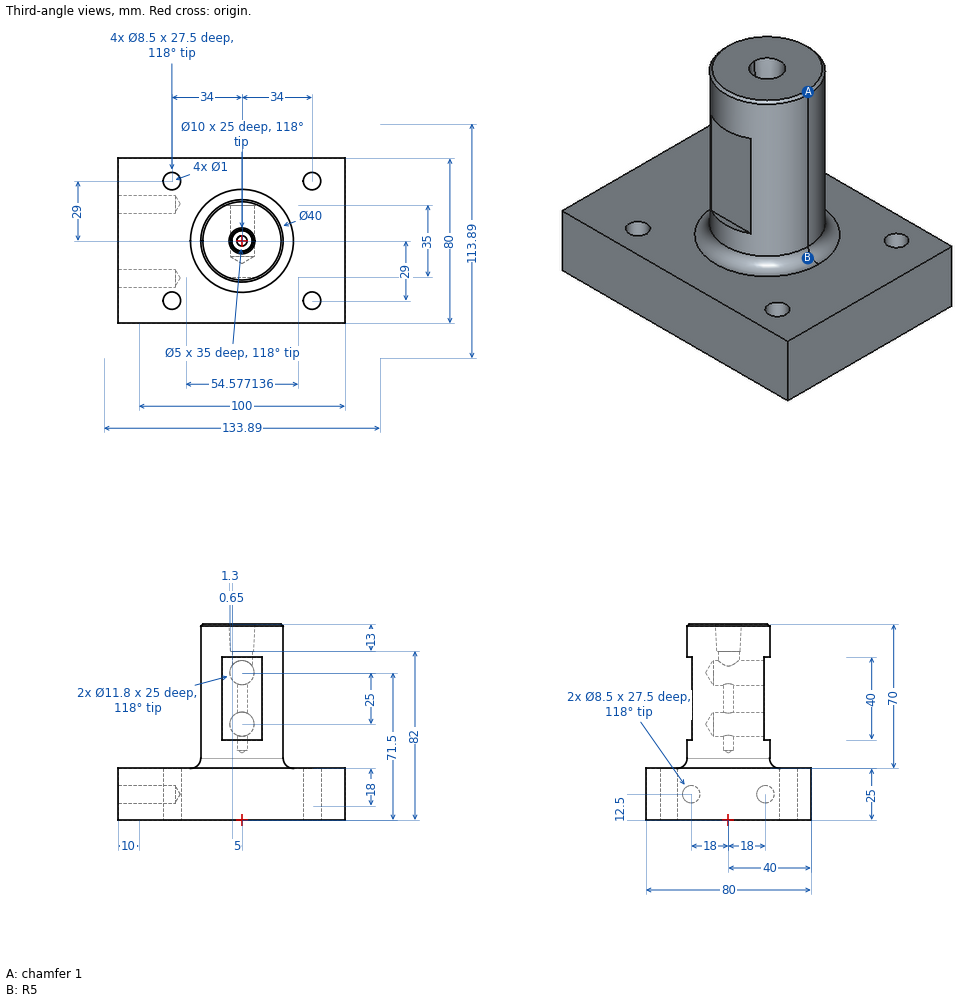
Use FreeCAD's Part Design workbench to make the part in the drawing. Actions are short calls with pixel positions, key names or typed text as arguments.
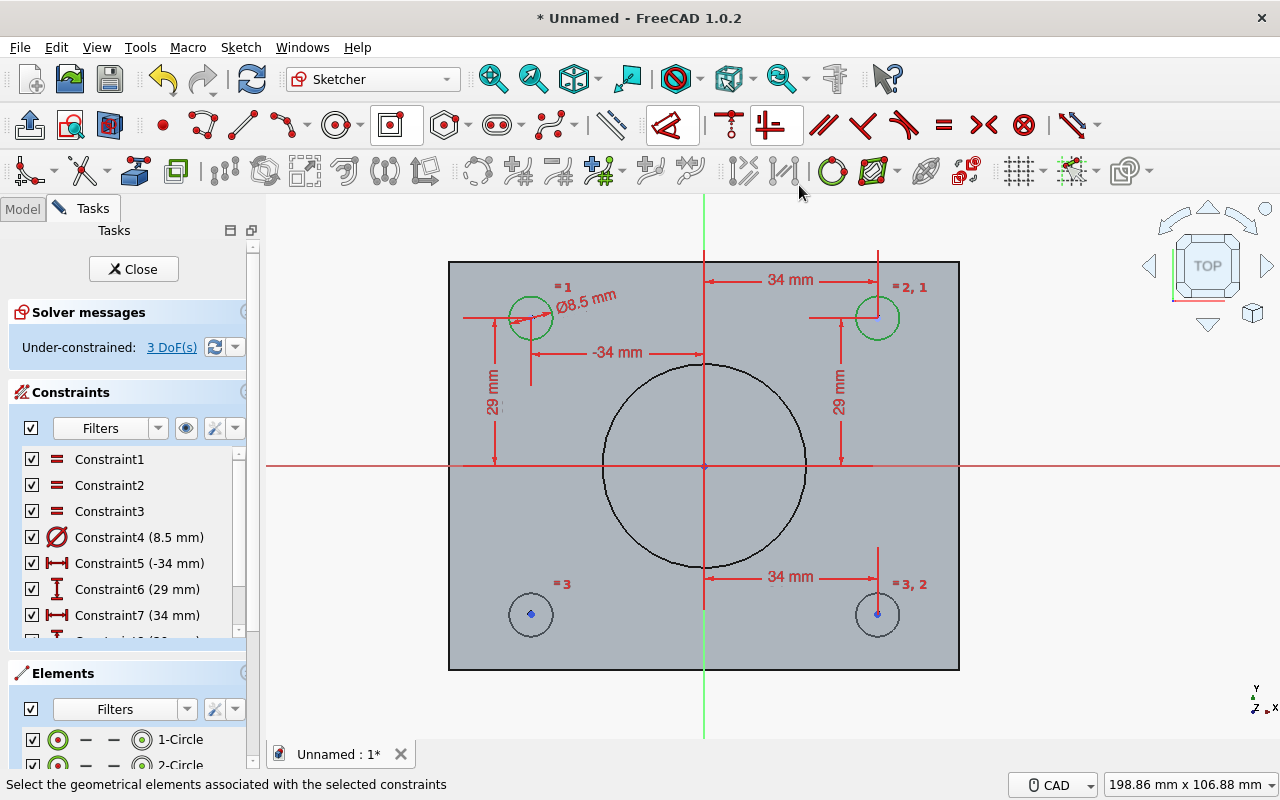
click(878, 615)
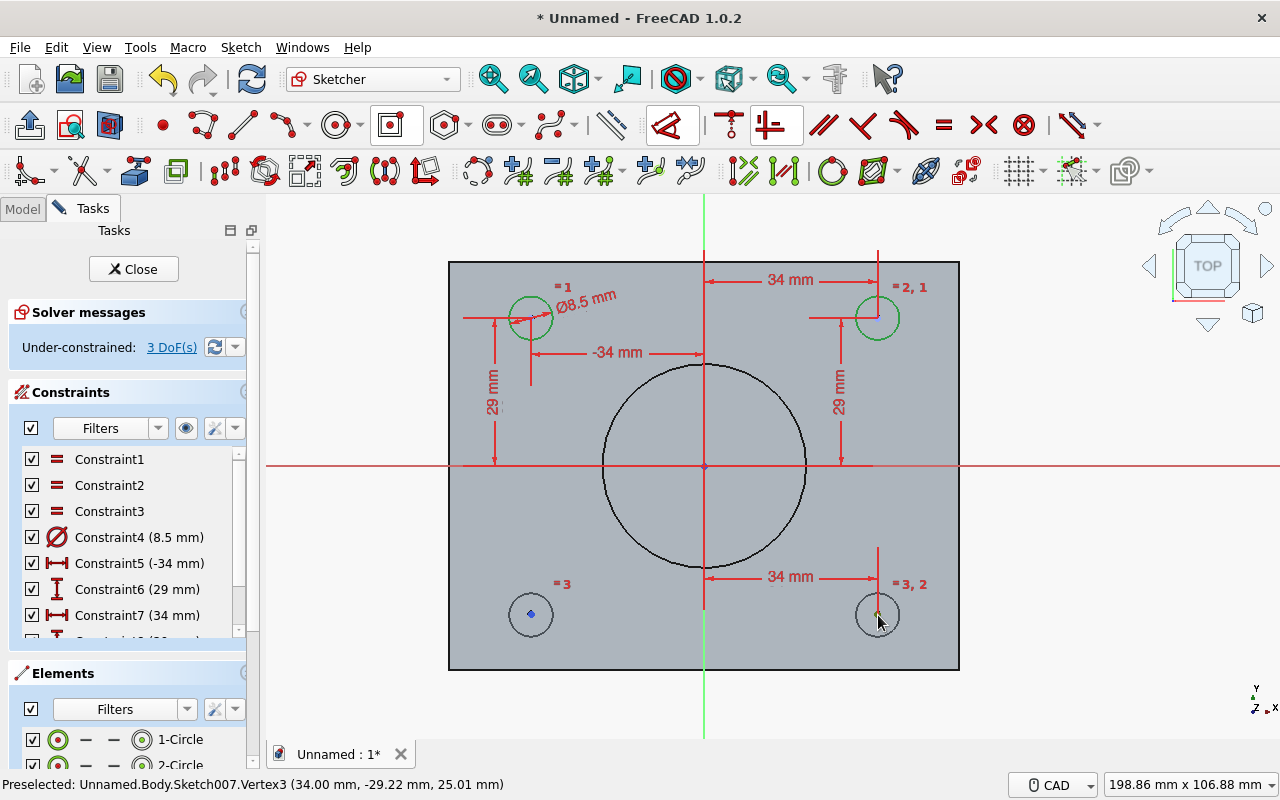
click(694, 126)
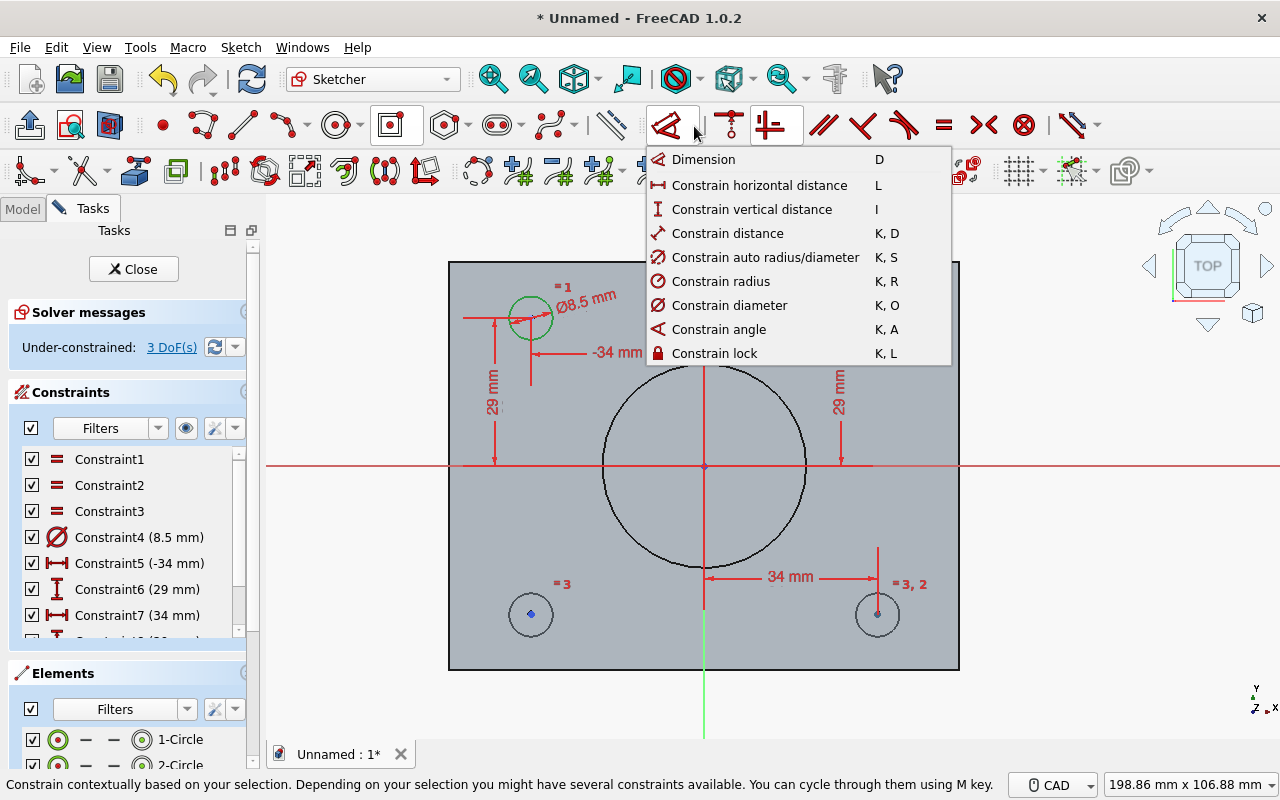
click(799, 209)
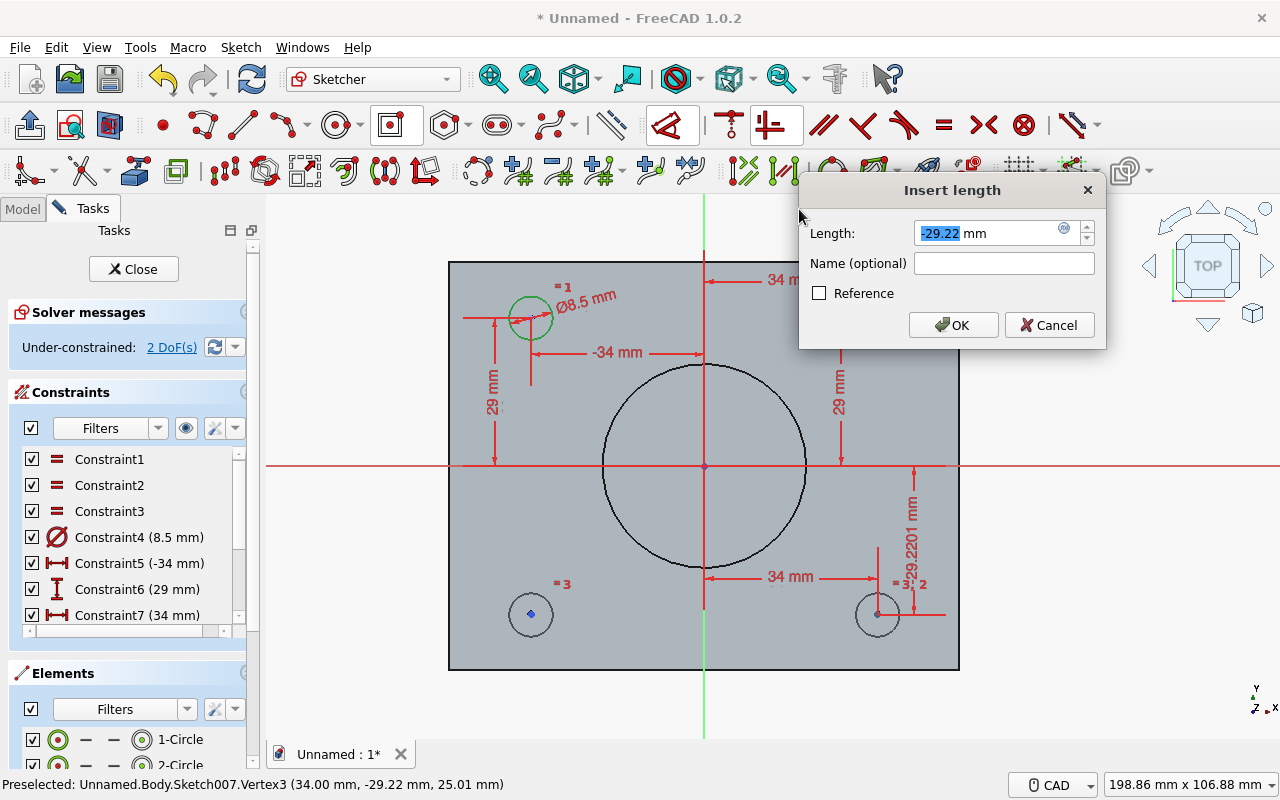
text(-29)
key(Return)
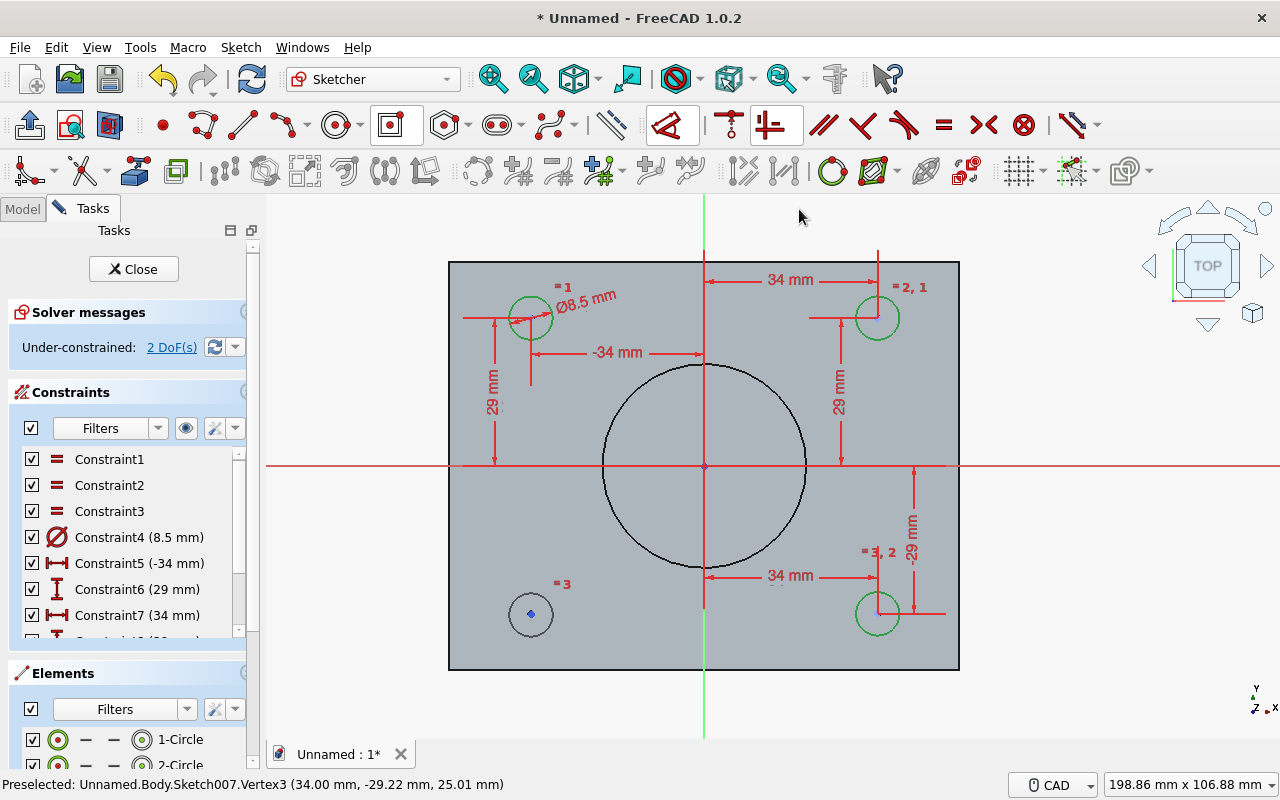
click(531, 615)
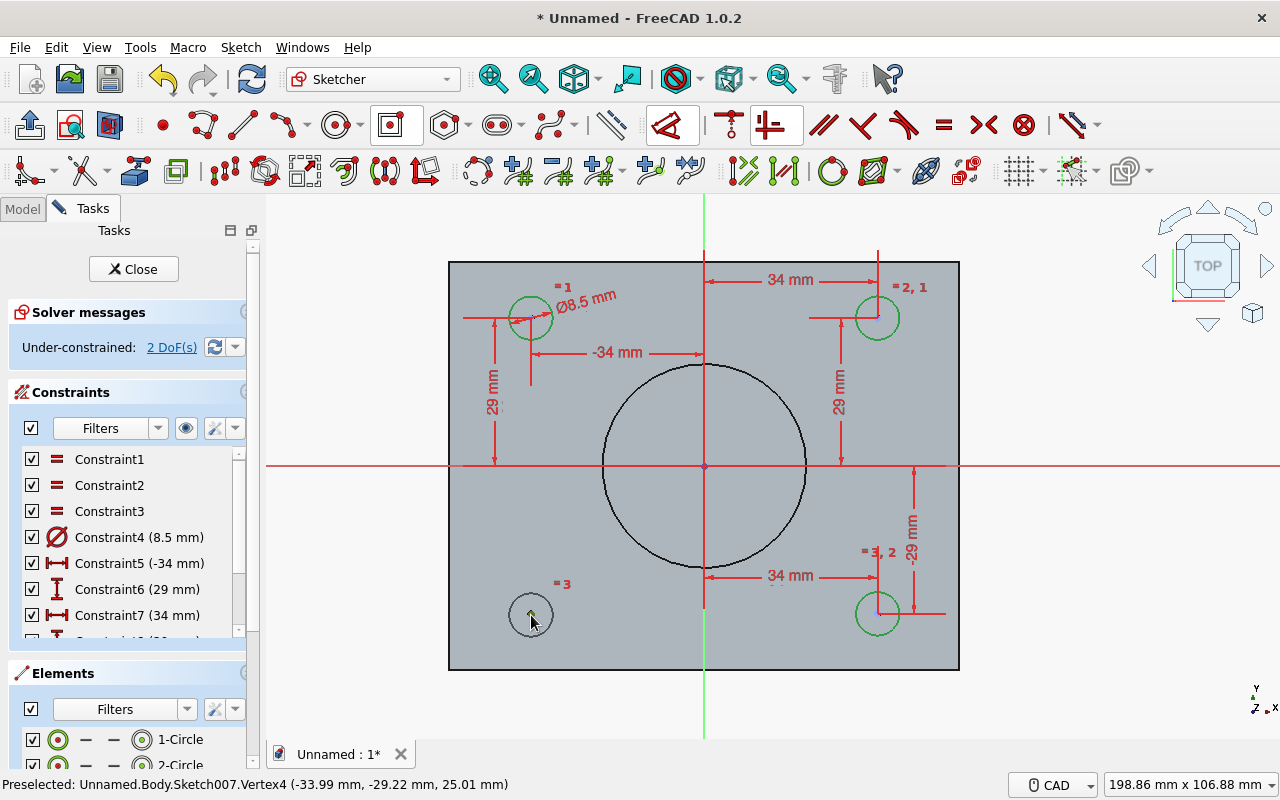
click(694, 126)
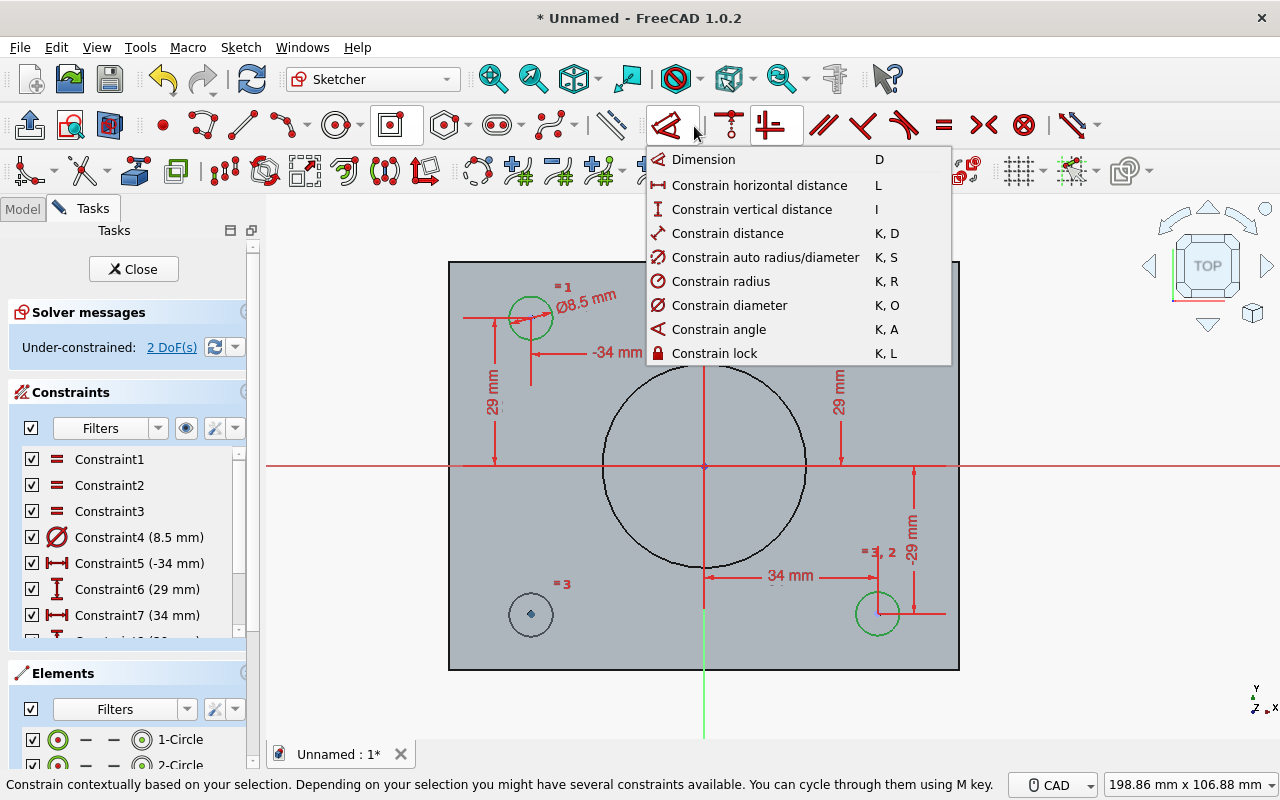
click(799, 185)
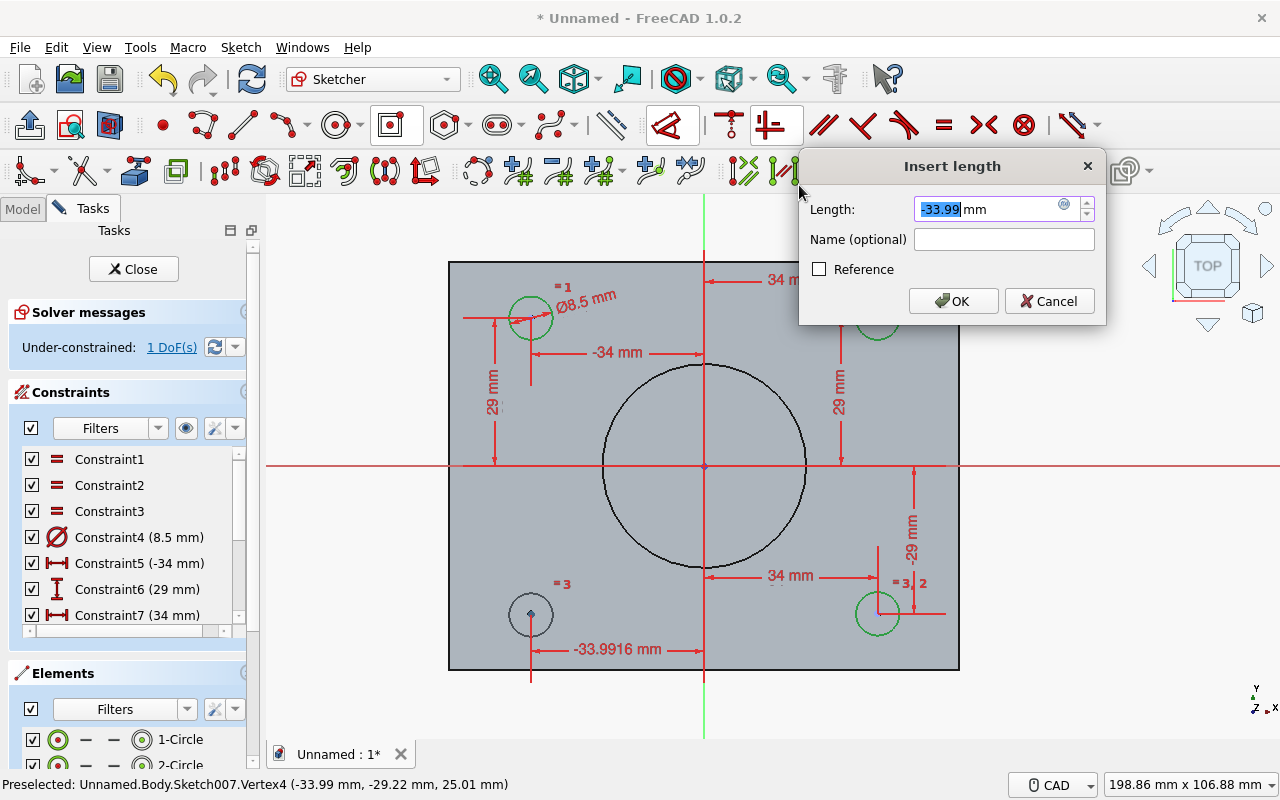
text(-34)
key(Return)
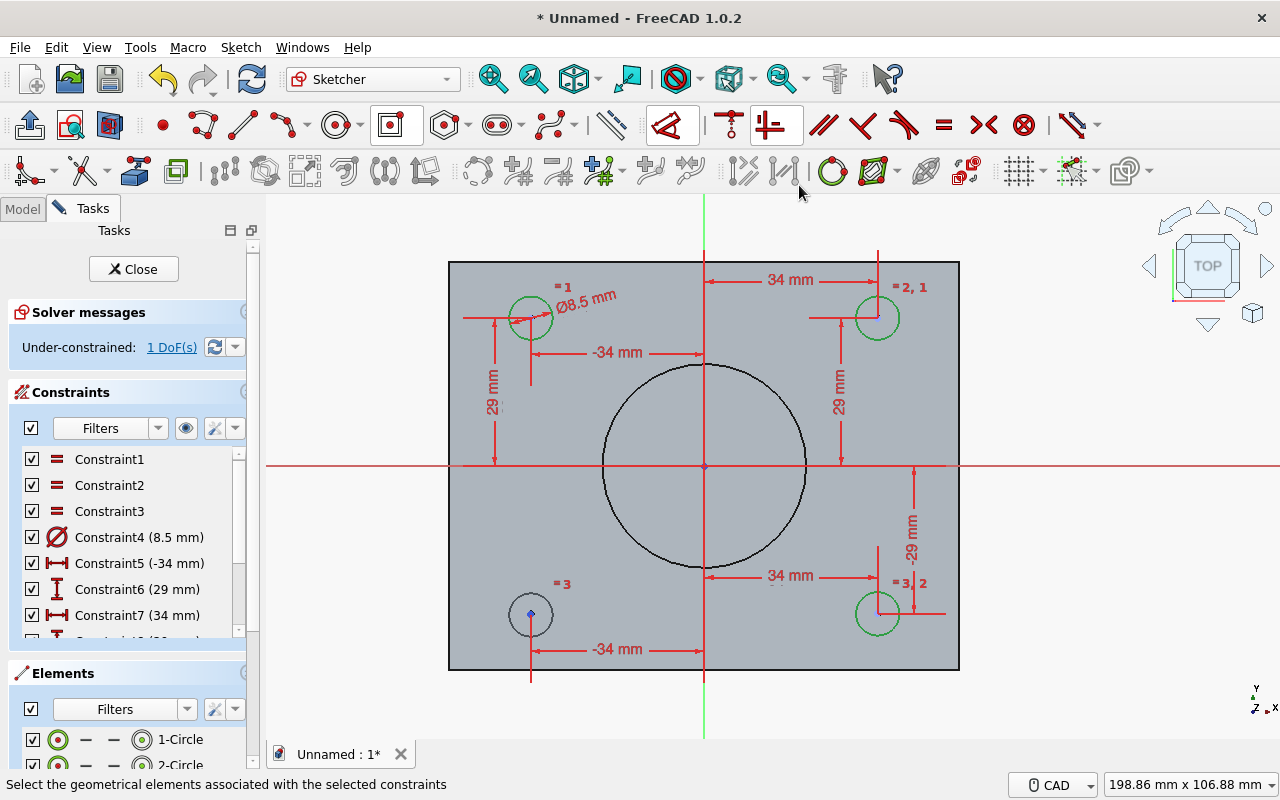
click(531, 615)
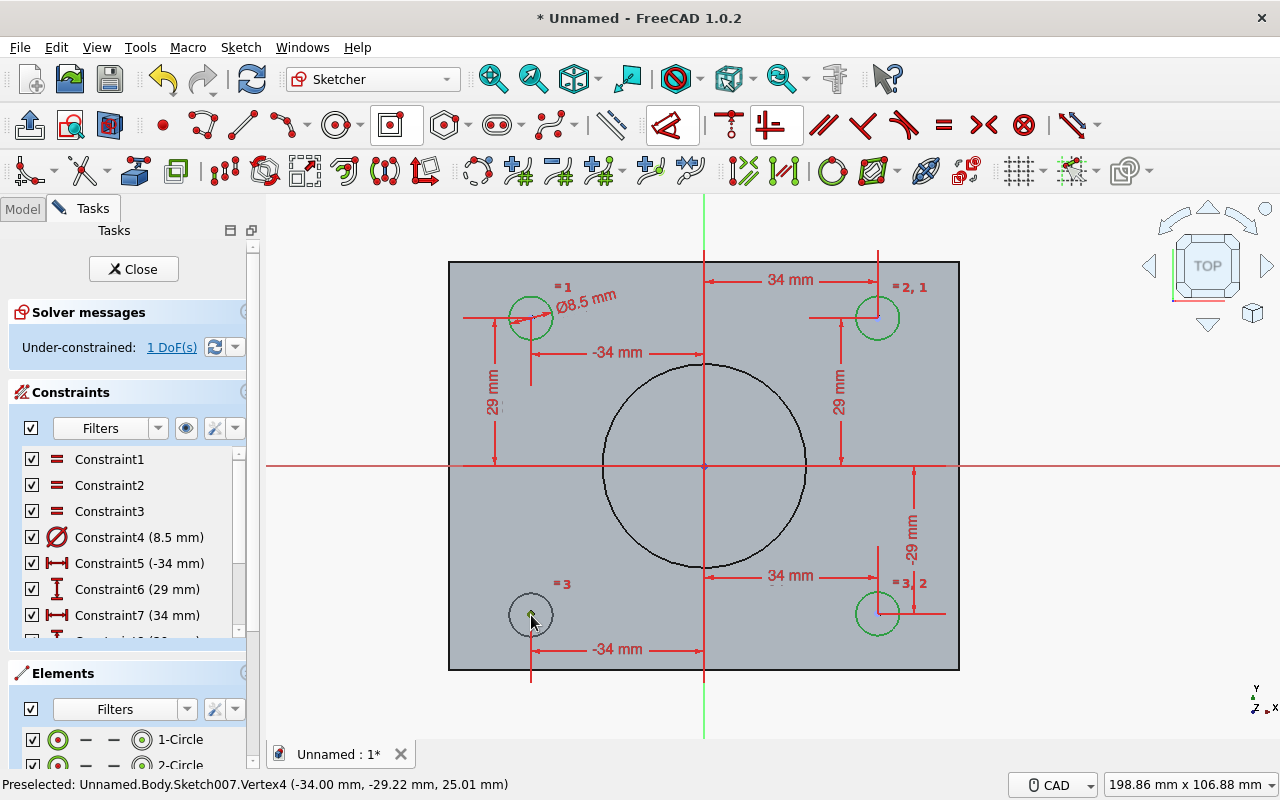
key(i)